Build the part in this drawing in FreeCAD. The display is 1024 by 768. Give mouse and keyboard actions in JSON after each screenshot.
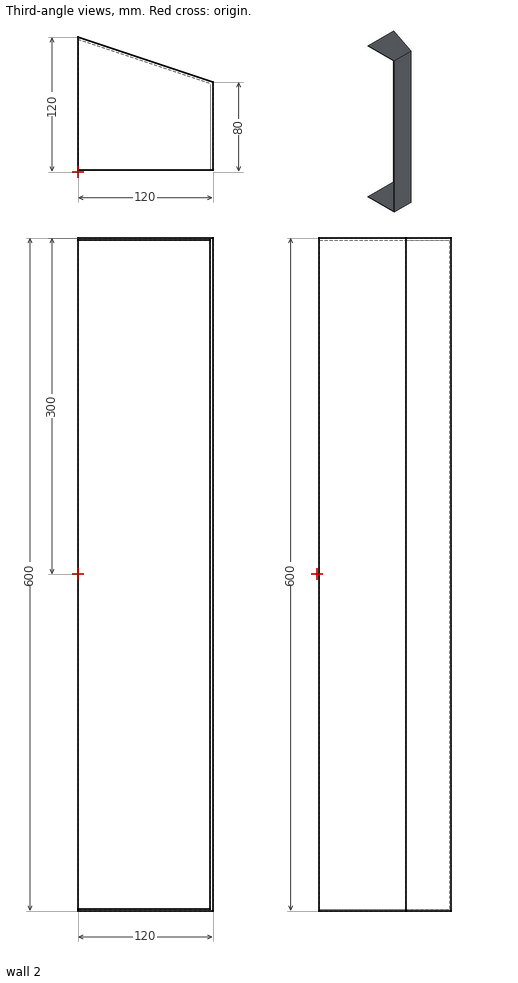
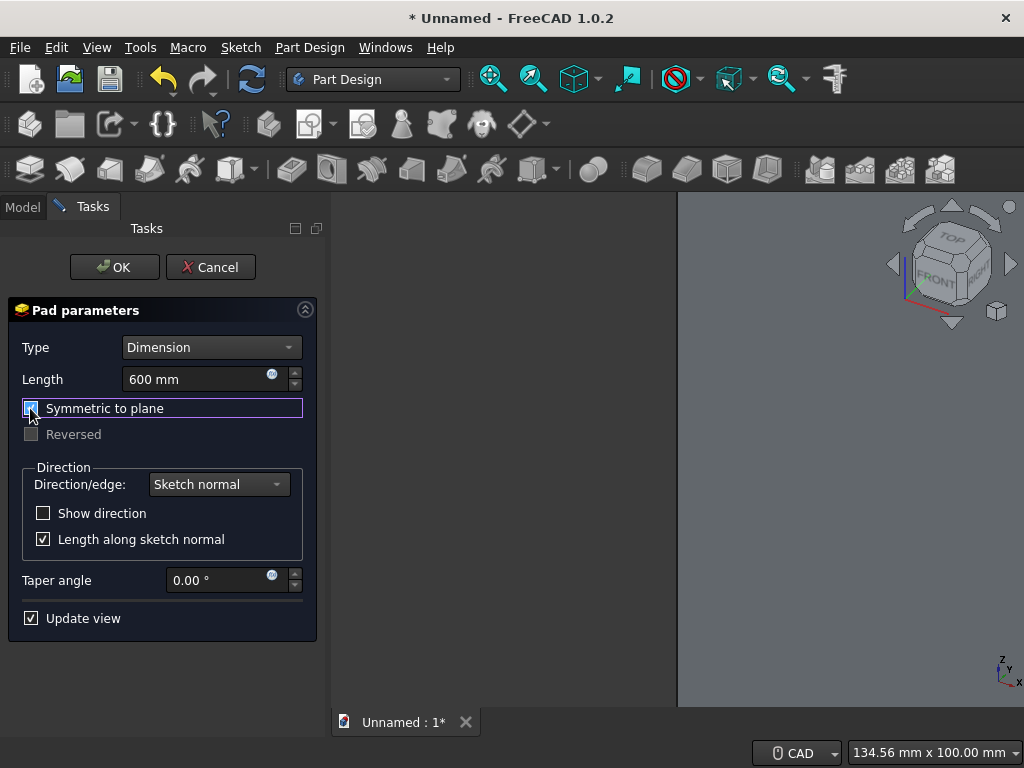
{"action": "left_click", "coordinate": [115, 267]}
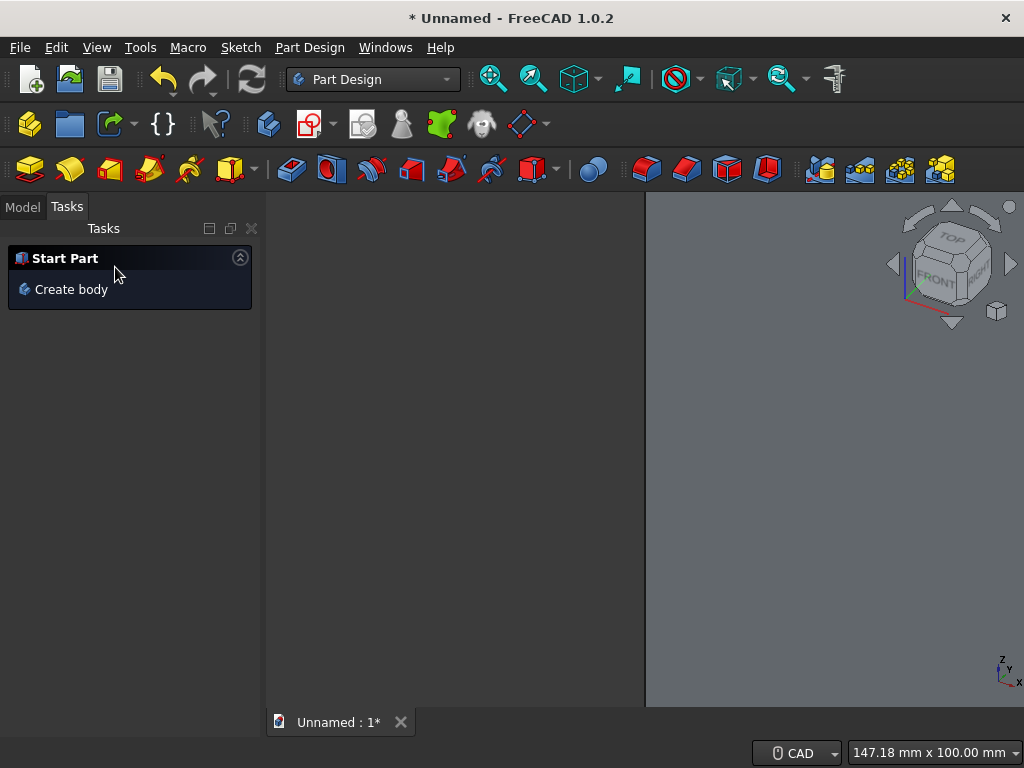
{"action": "left_click", "coordinate": [494, 80]}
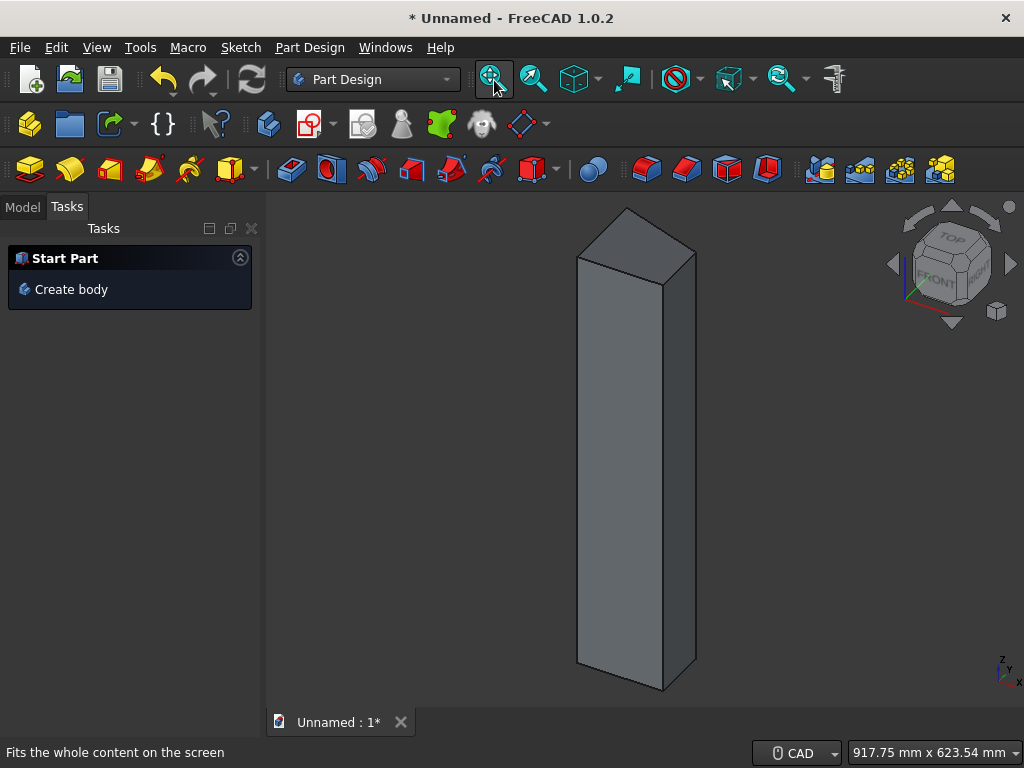
{"action": "key", "text": "0"}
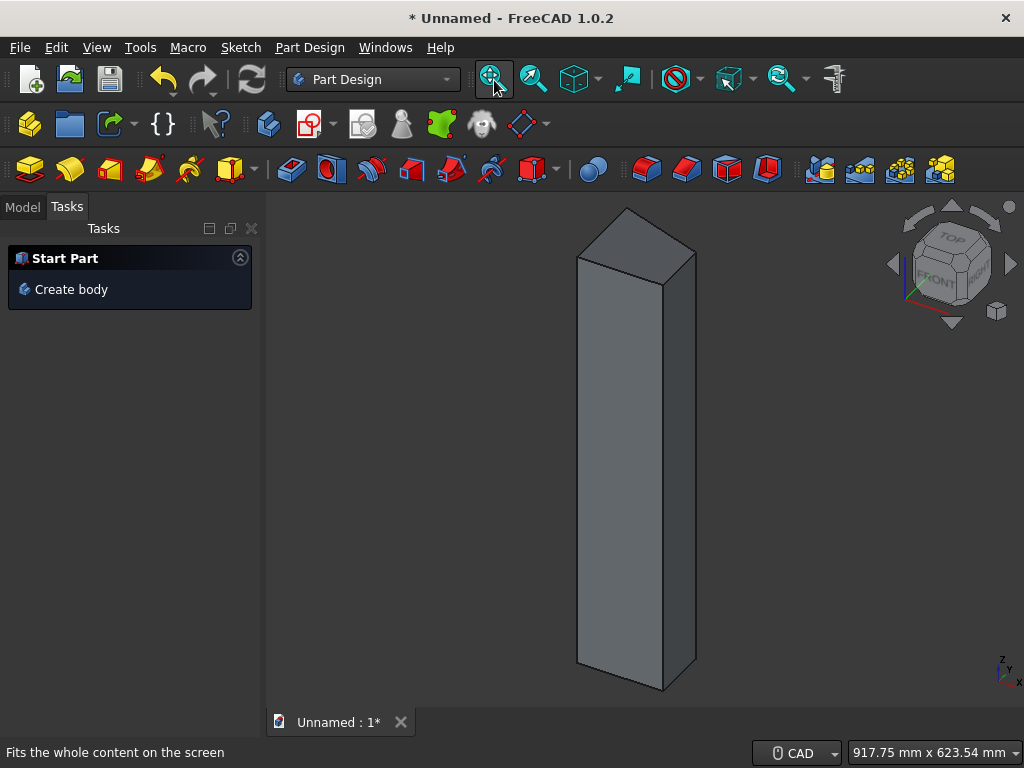
{"action": "key", "text": "2"}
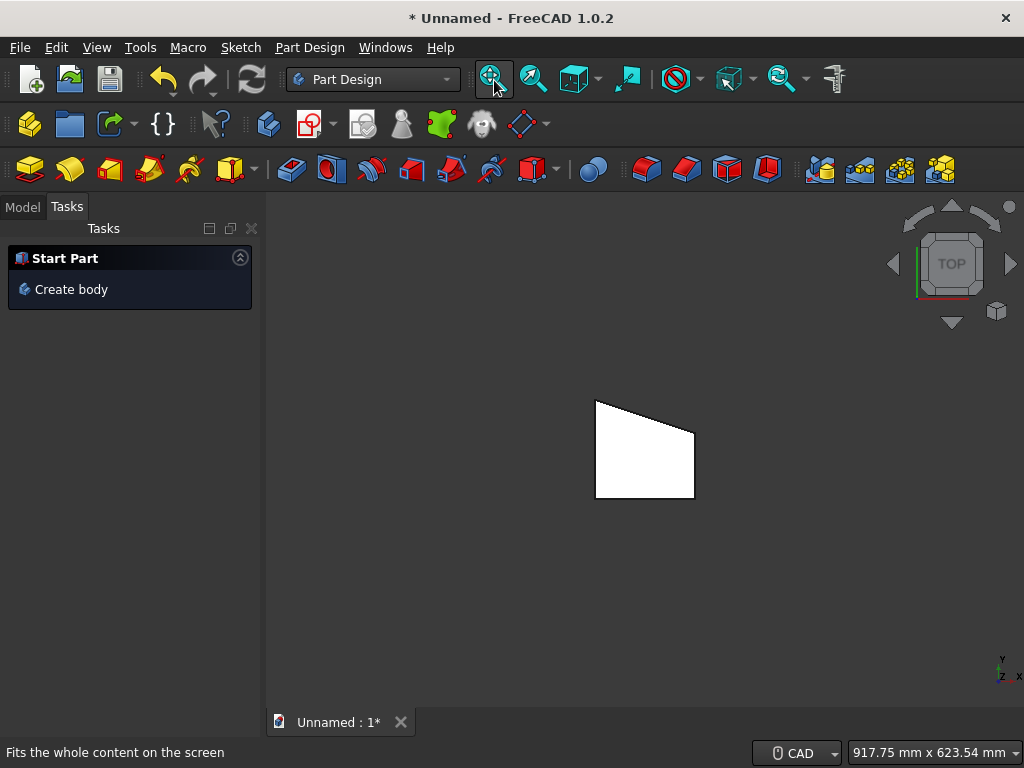
{"action": "left_click", "coordinate": [494, 80]}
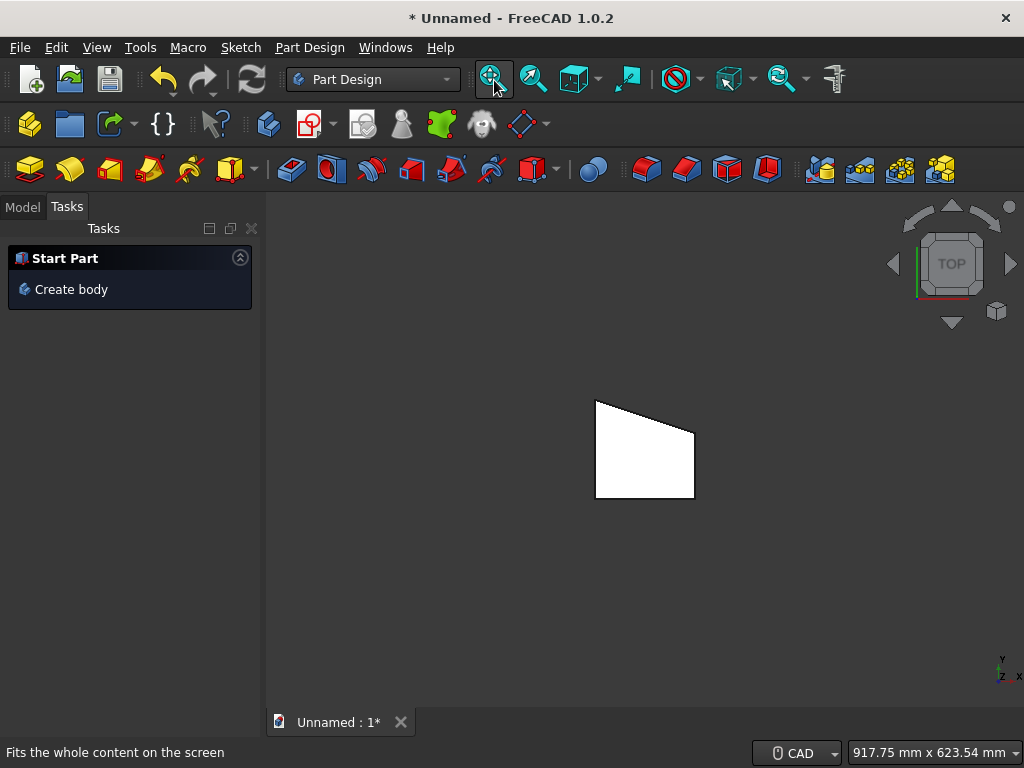
{"action": "key", "text": "1"}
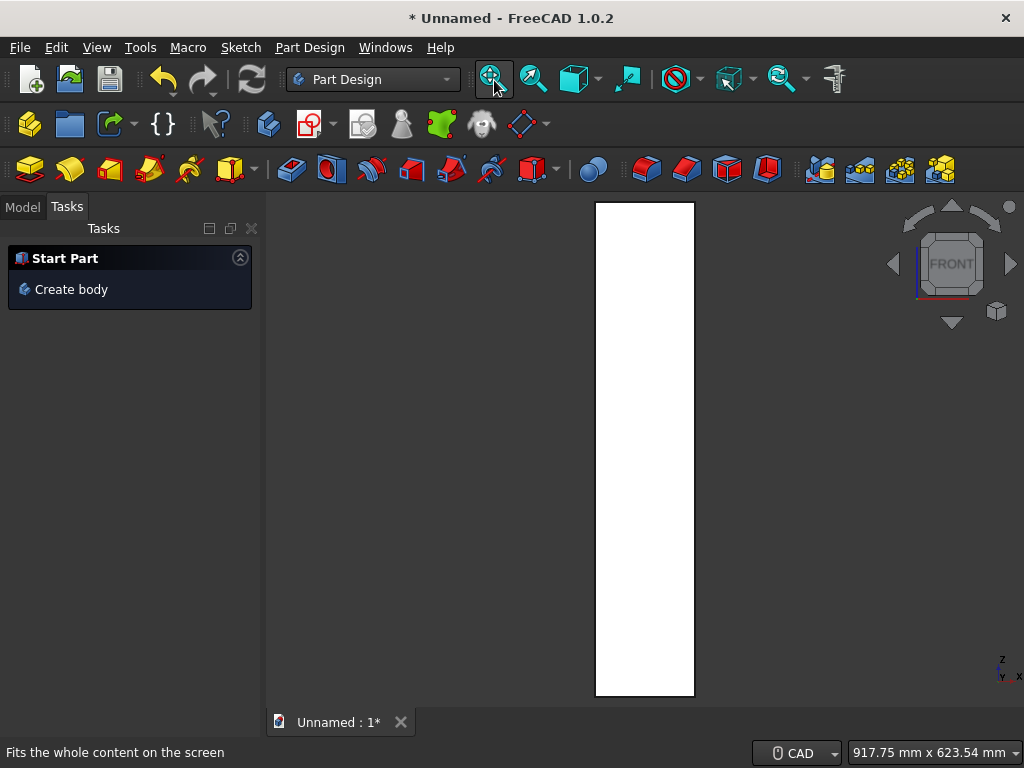
{"action": "key", "text": "3"}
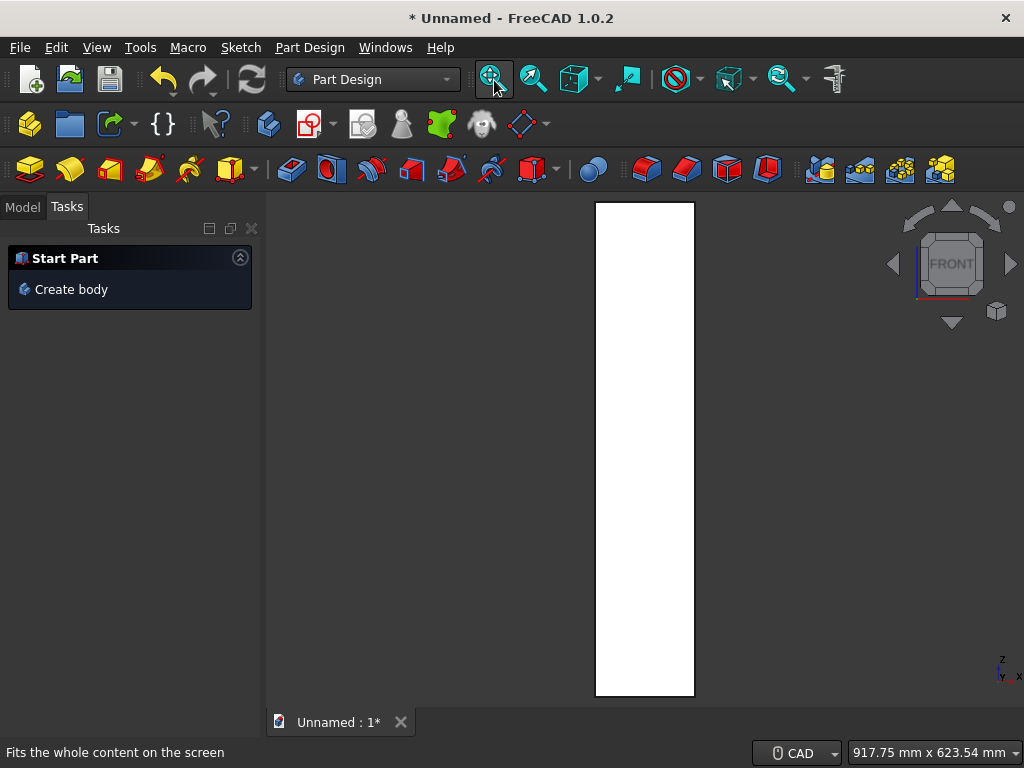
{"action": "key", "text": "5"}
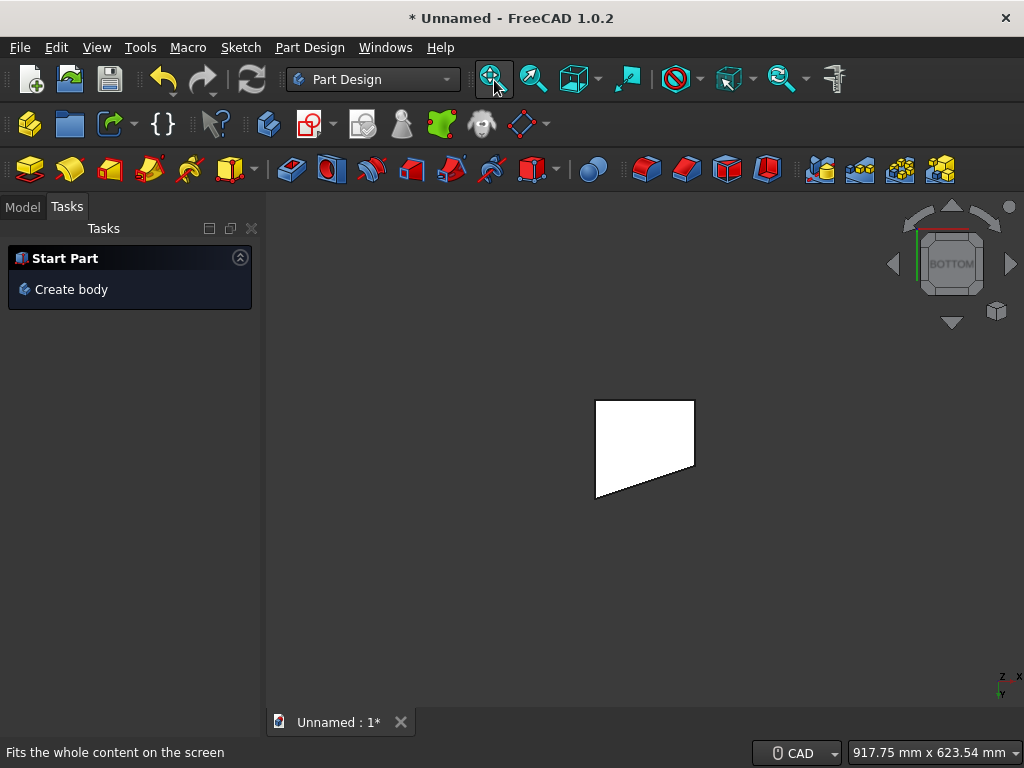
{"action": "left_click", "coordinate": [494, 80]}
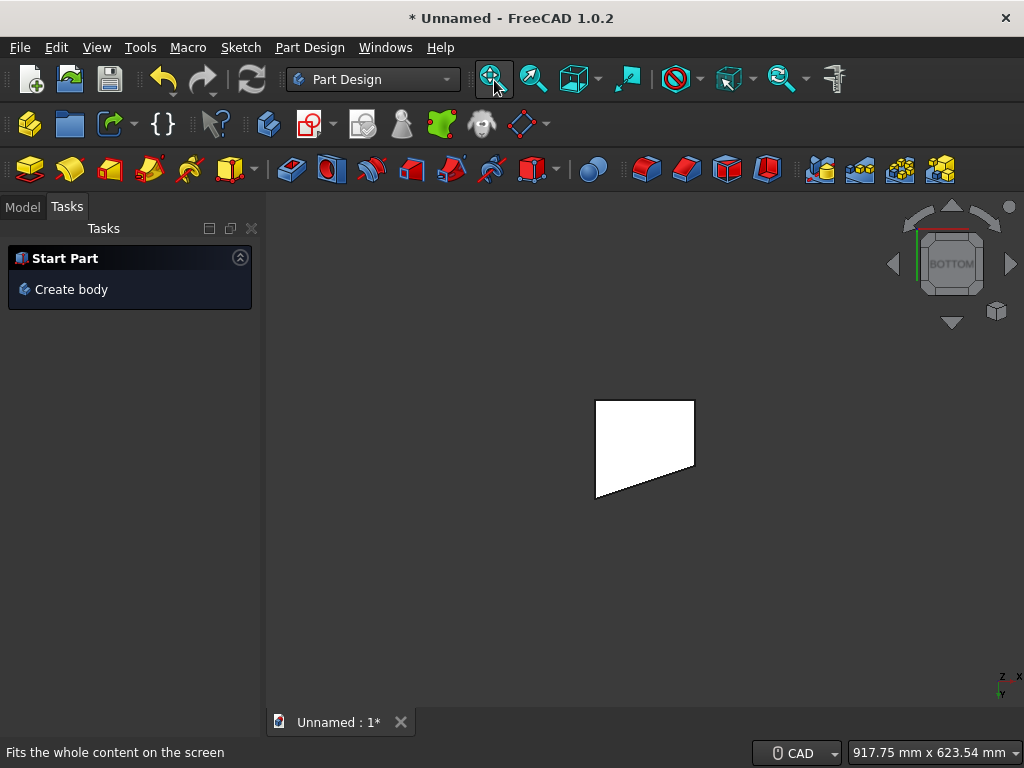
{"action": "key", "text": "4"}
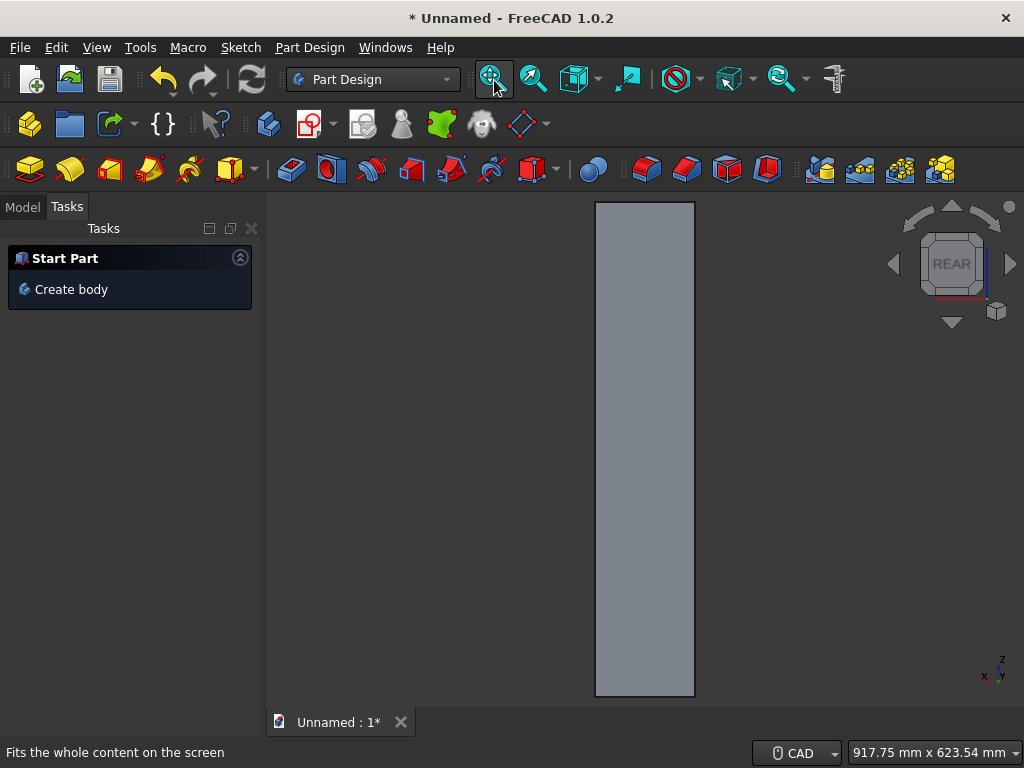
{"action": "key", "text": "6"}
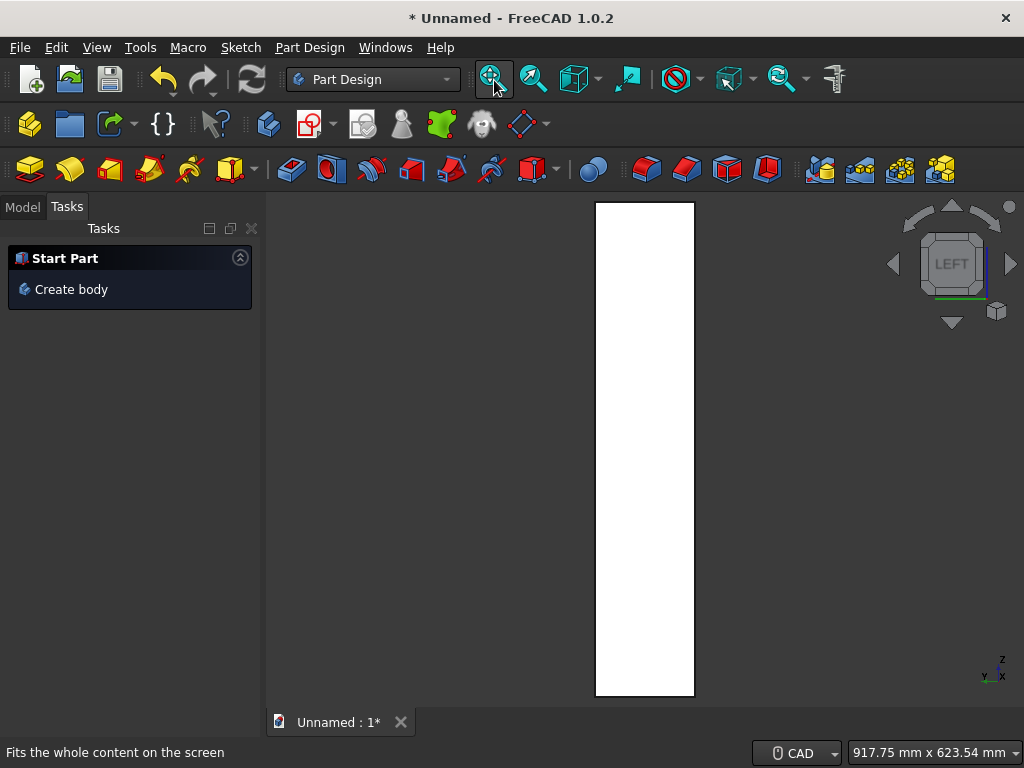
{"action": "left_click", "coordinate": [645, 307]}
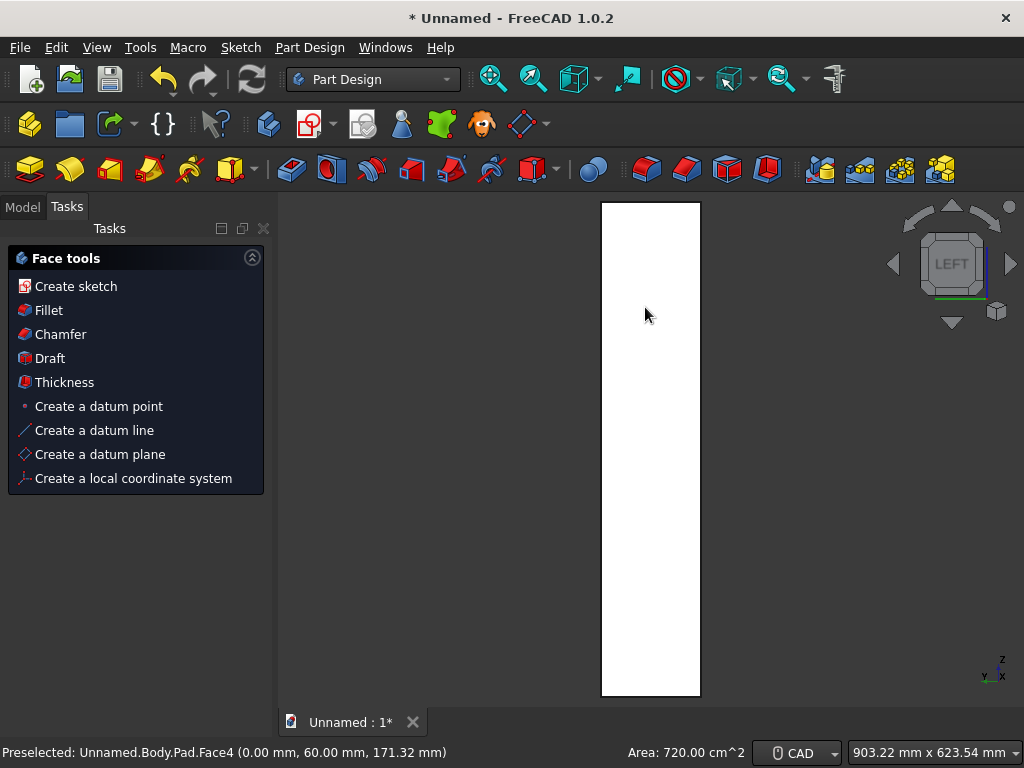
{"action": "left_click", "coordinate": [768, 170]}